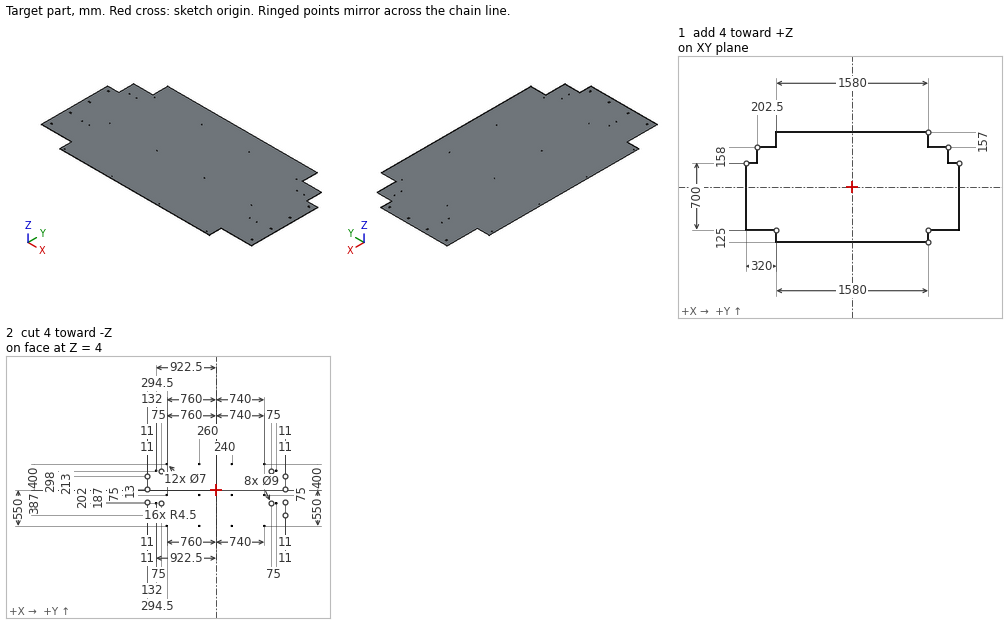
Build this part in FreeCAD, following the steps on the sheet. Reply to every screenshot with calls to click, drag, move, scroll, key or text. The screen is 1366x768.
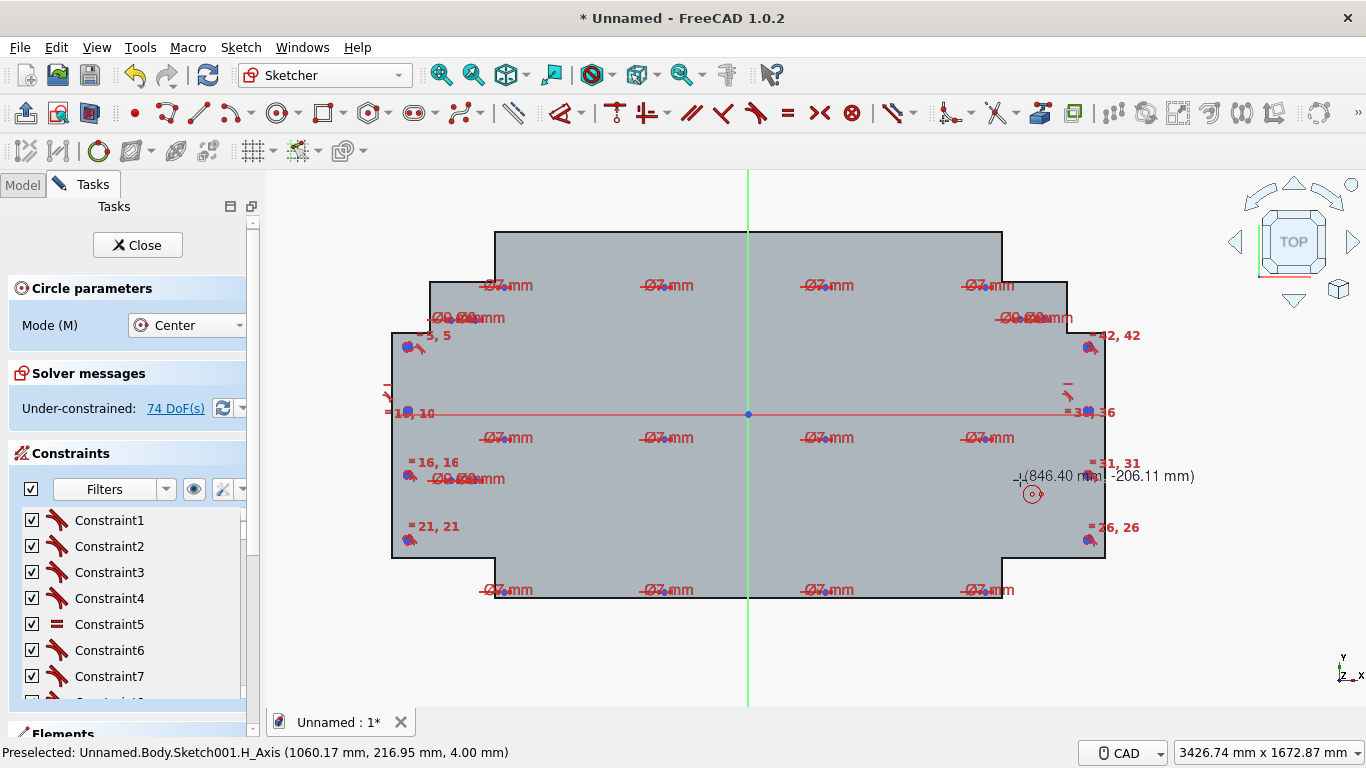
click(1020, 480)
move(1021, 479)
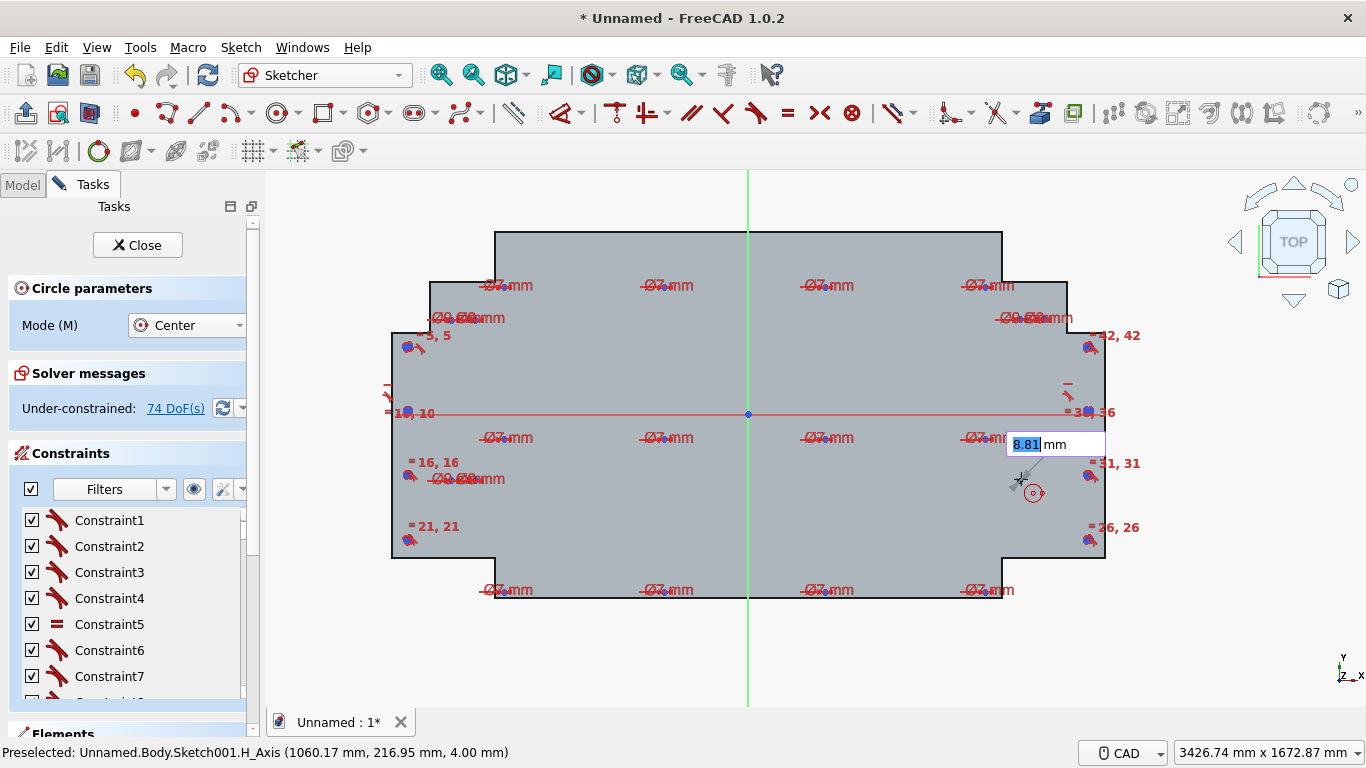
text(9)
key(Return)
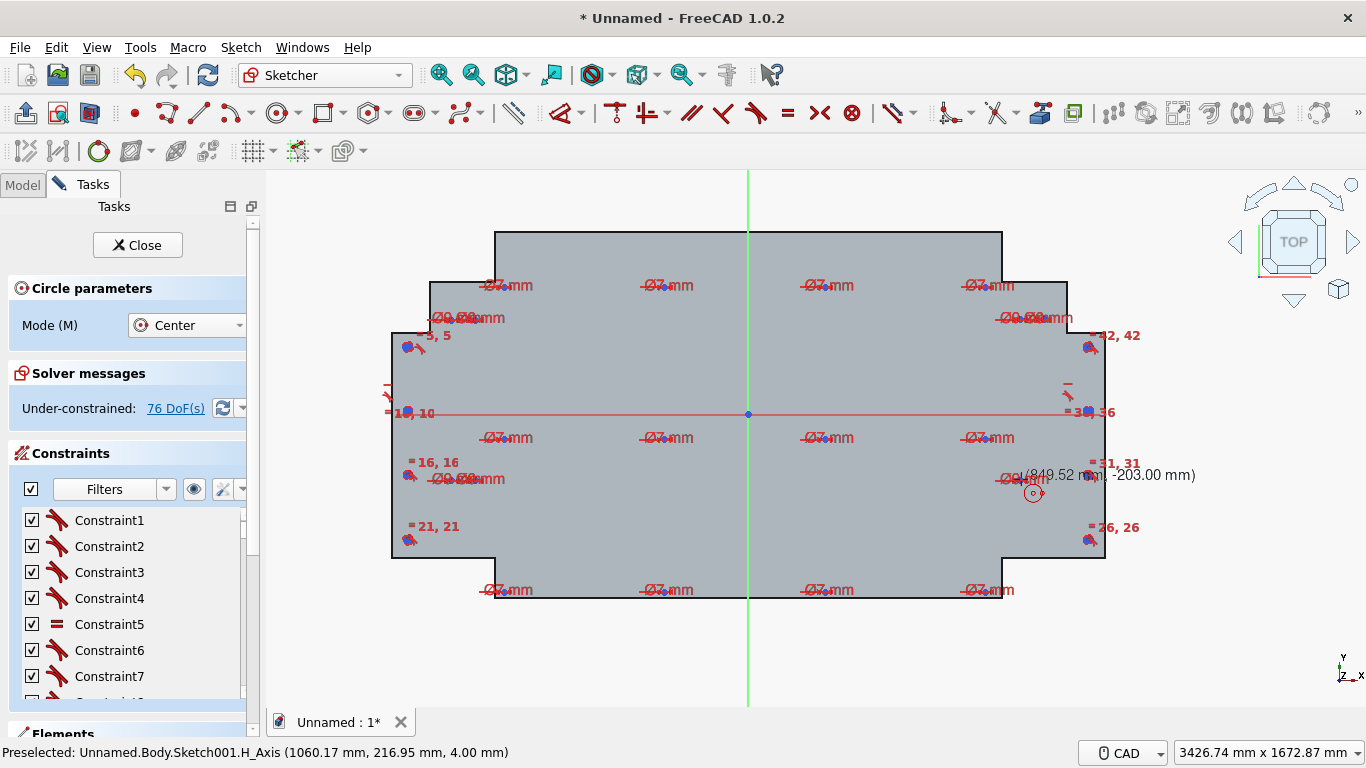
scroll(1044, 480, up, 14)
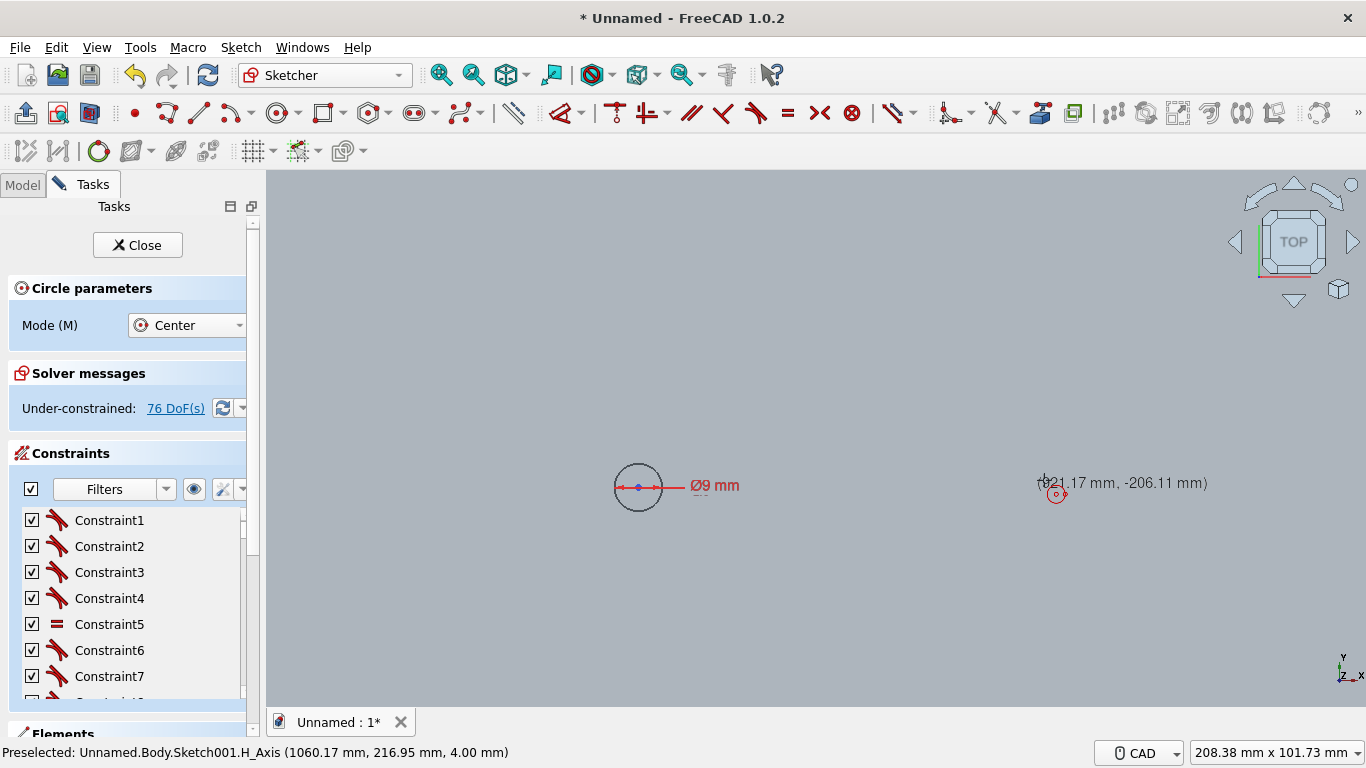
scroll(1044, 480, down, 14)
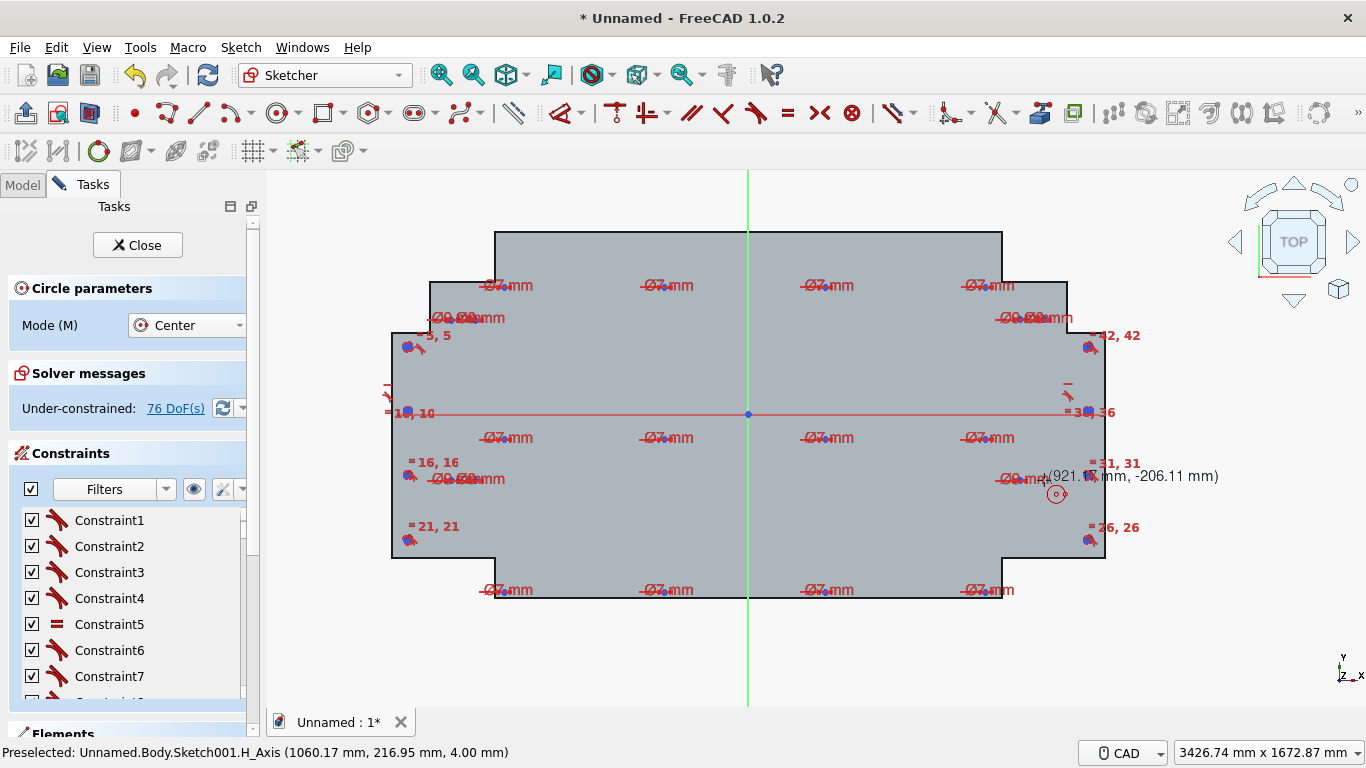
click(1044, 480)
move(1045, 479)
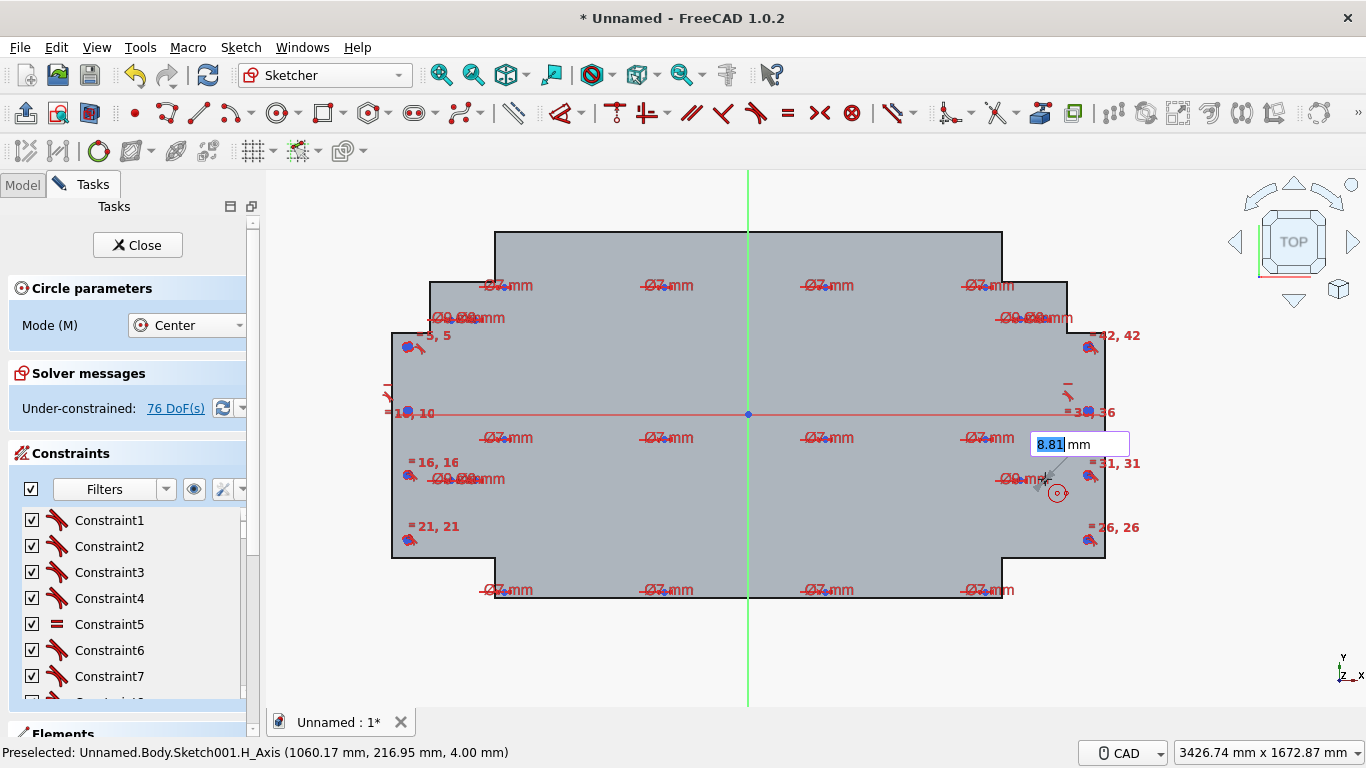
text(9)
key(Return)
key(Escape)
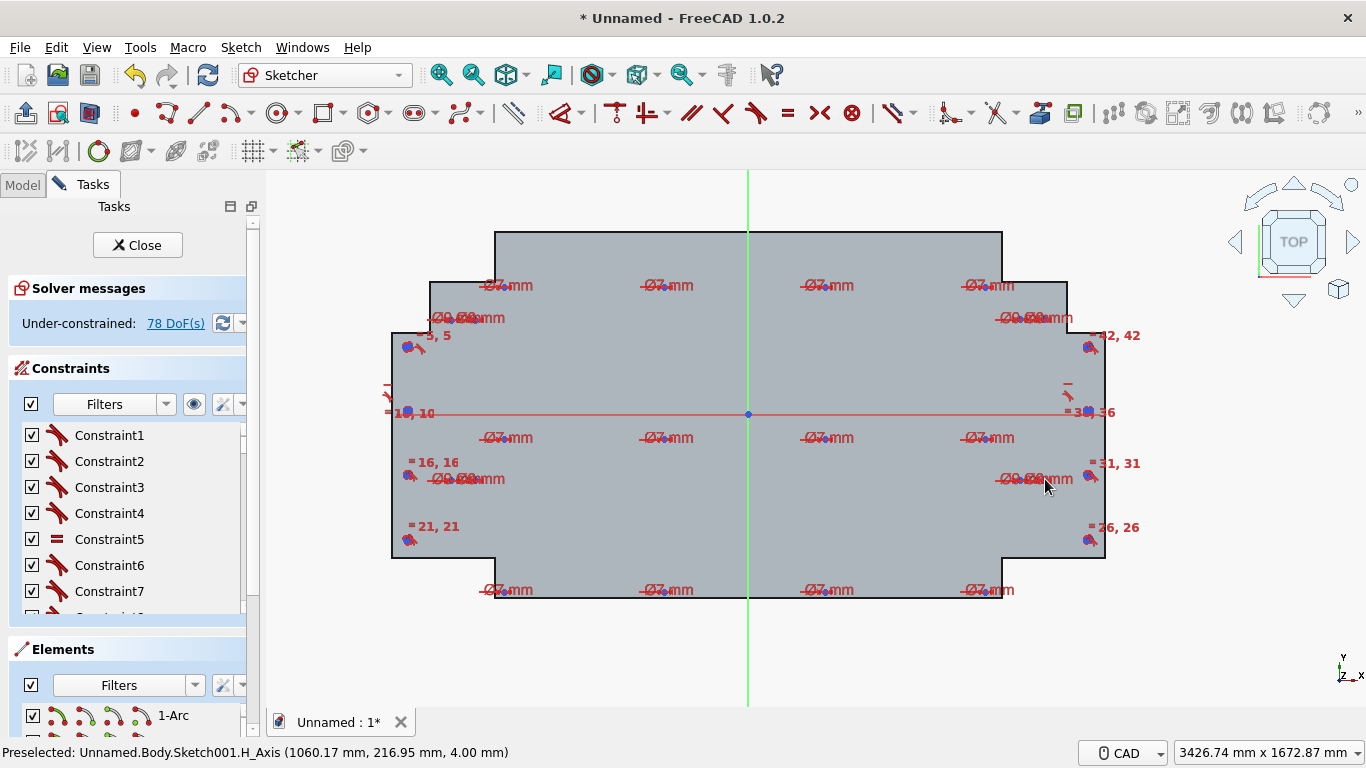
scroll(408, 345, up, 10)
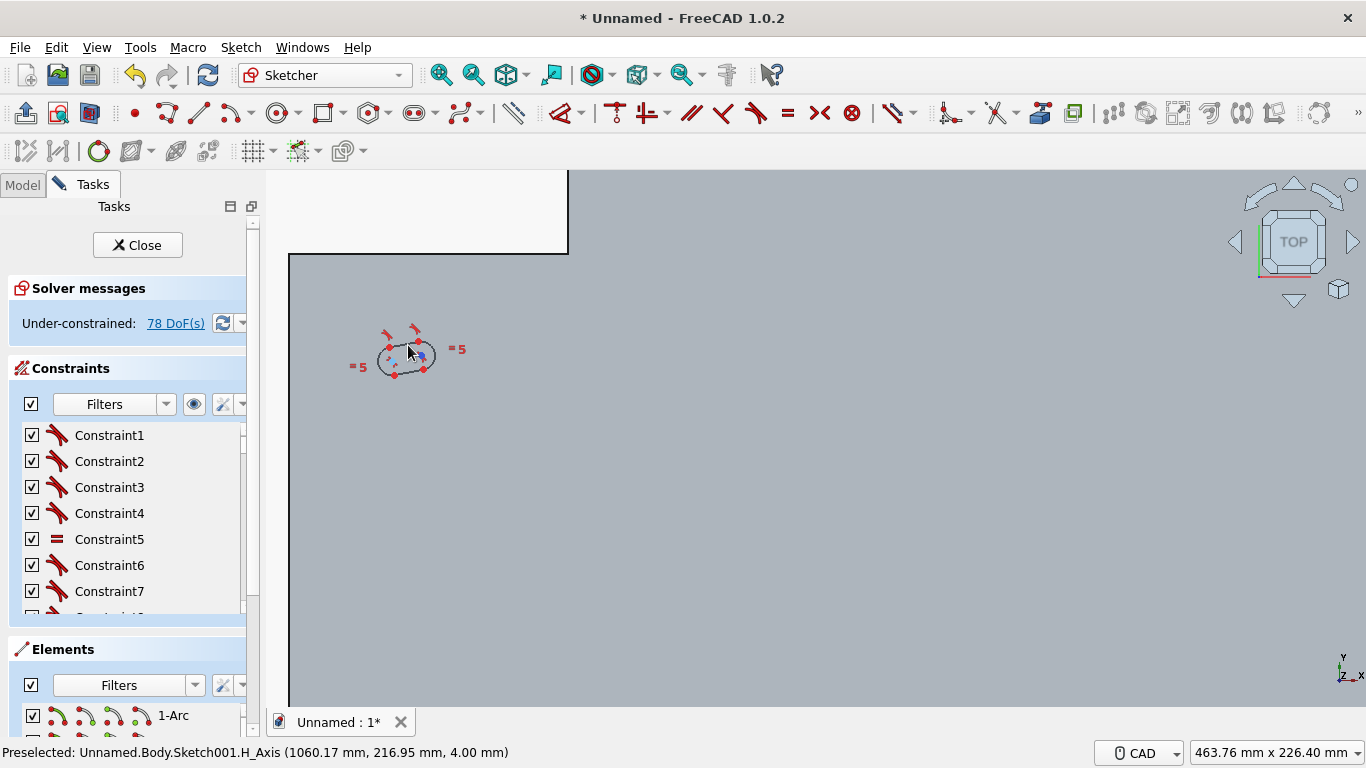
click(404, 345)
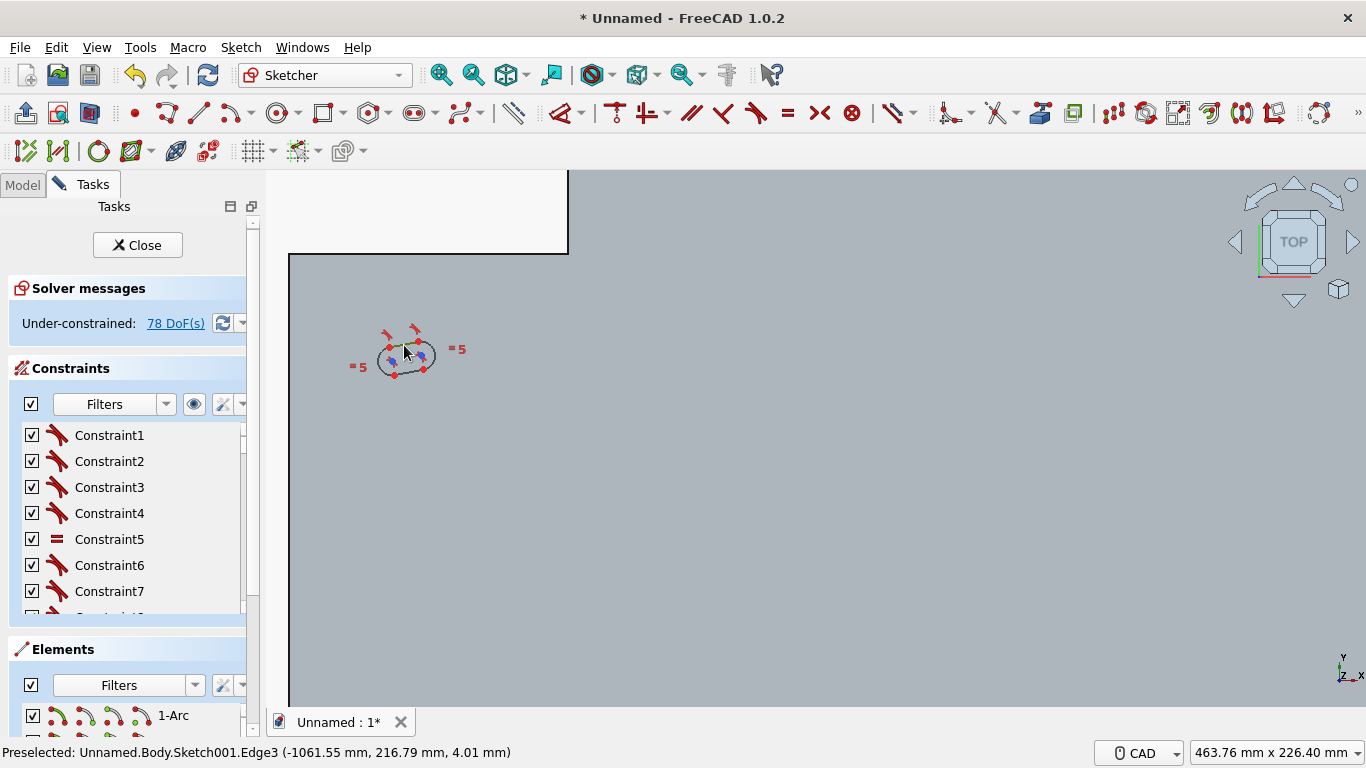
click(670, 114)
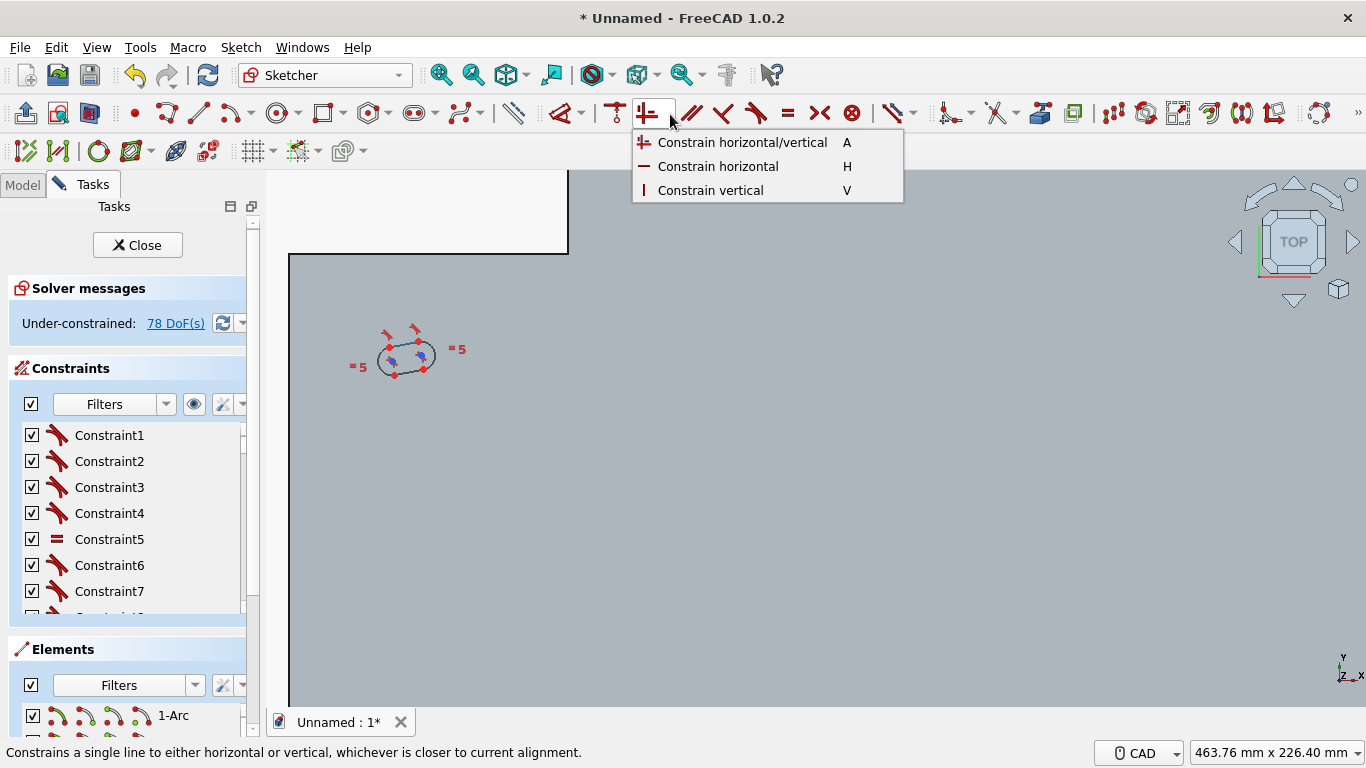
click(768, 166)